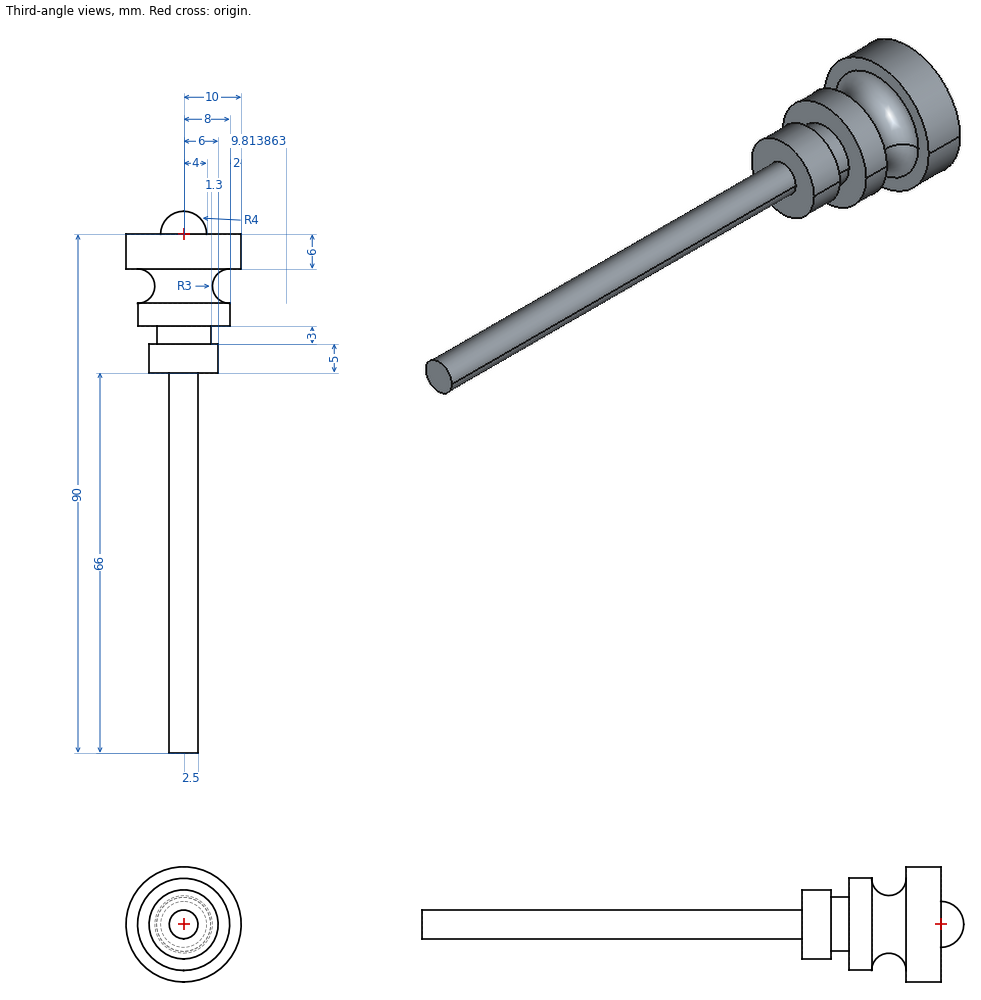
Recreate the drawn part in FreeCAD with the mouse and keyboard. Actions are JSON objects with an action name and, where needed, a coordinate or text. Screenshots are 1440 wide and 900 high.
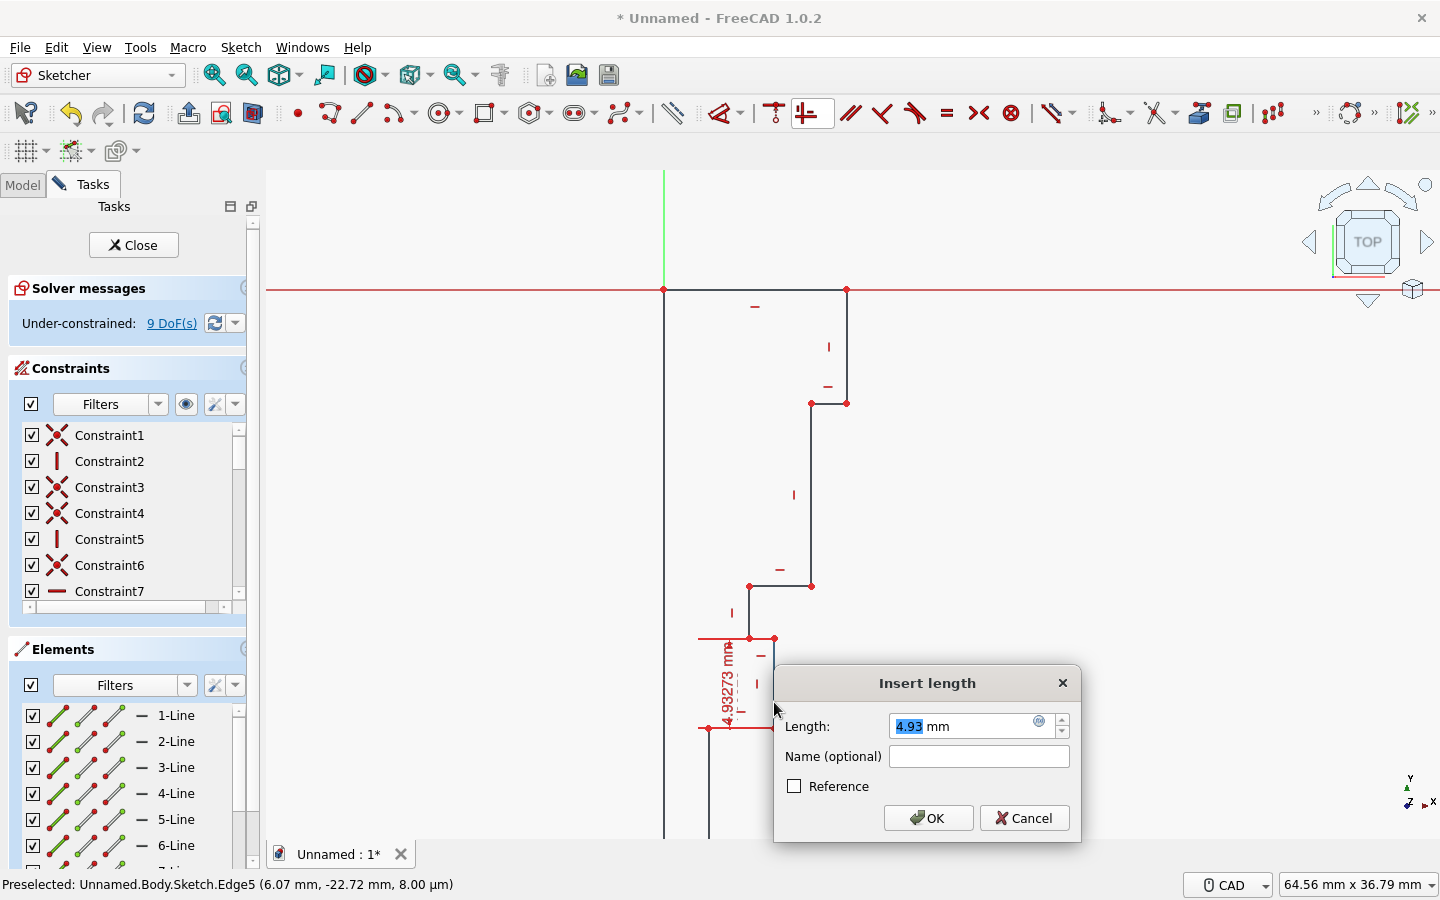
{"action": "type", "text": "5"}
{"action": "key", "text": "Return"}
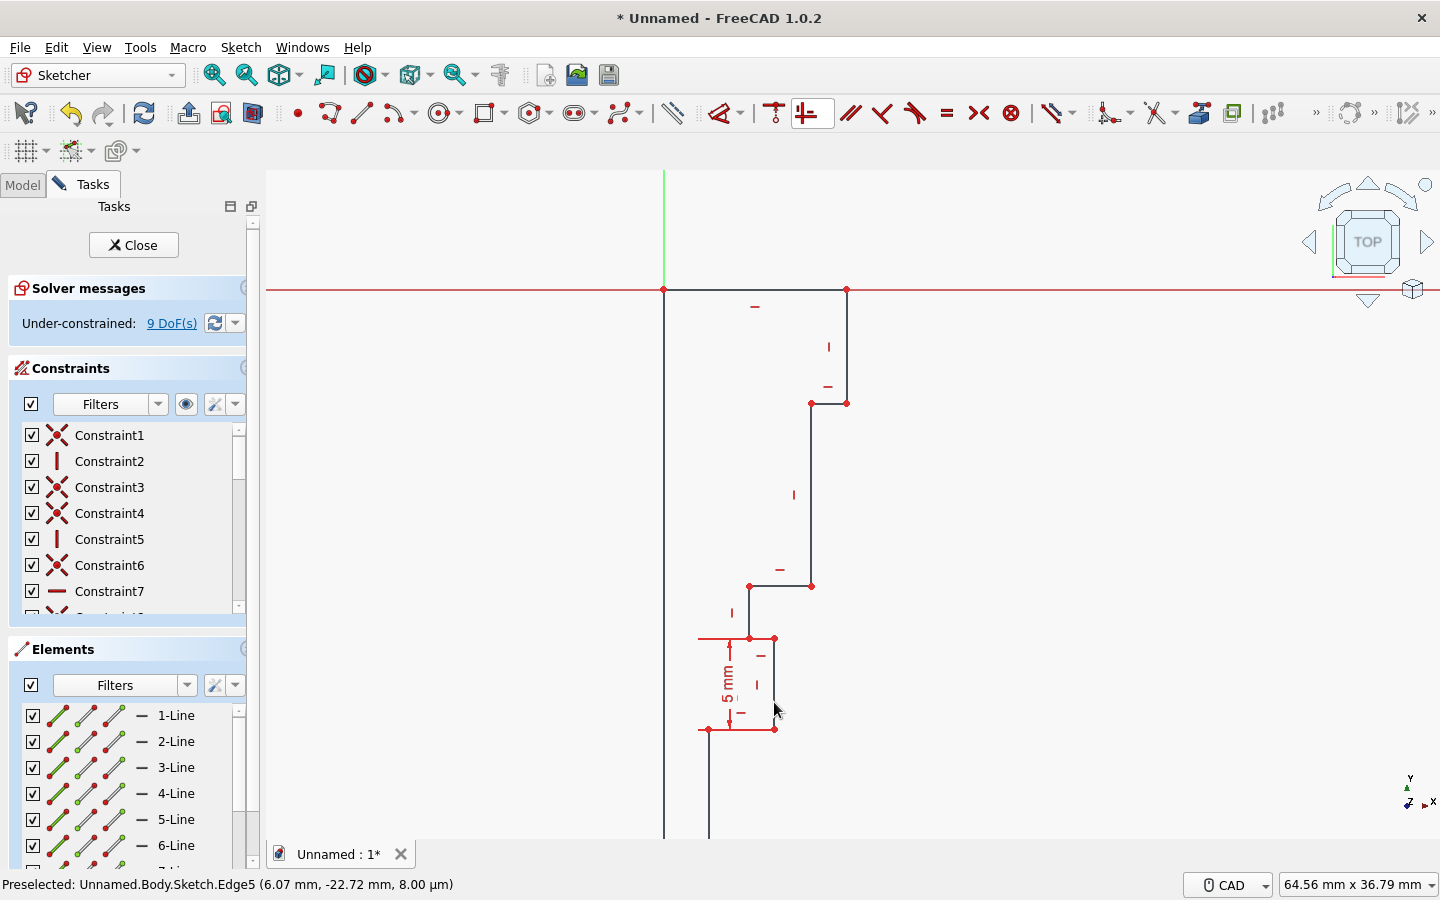
{"action": "left_click", "coordinate": [749, 623]}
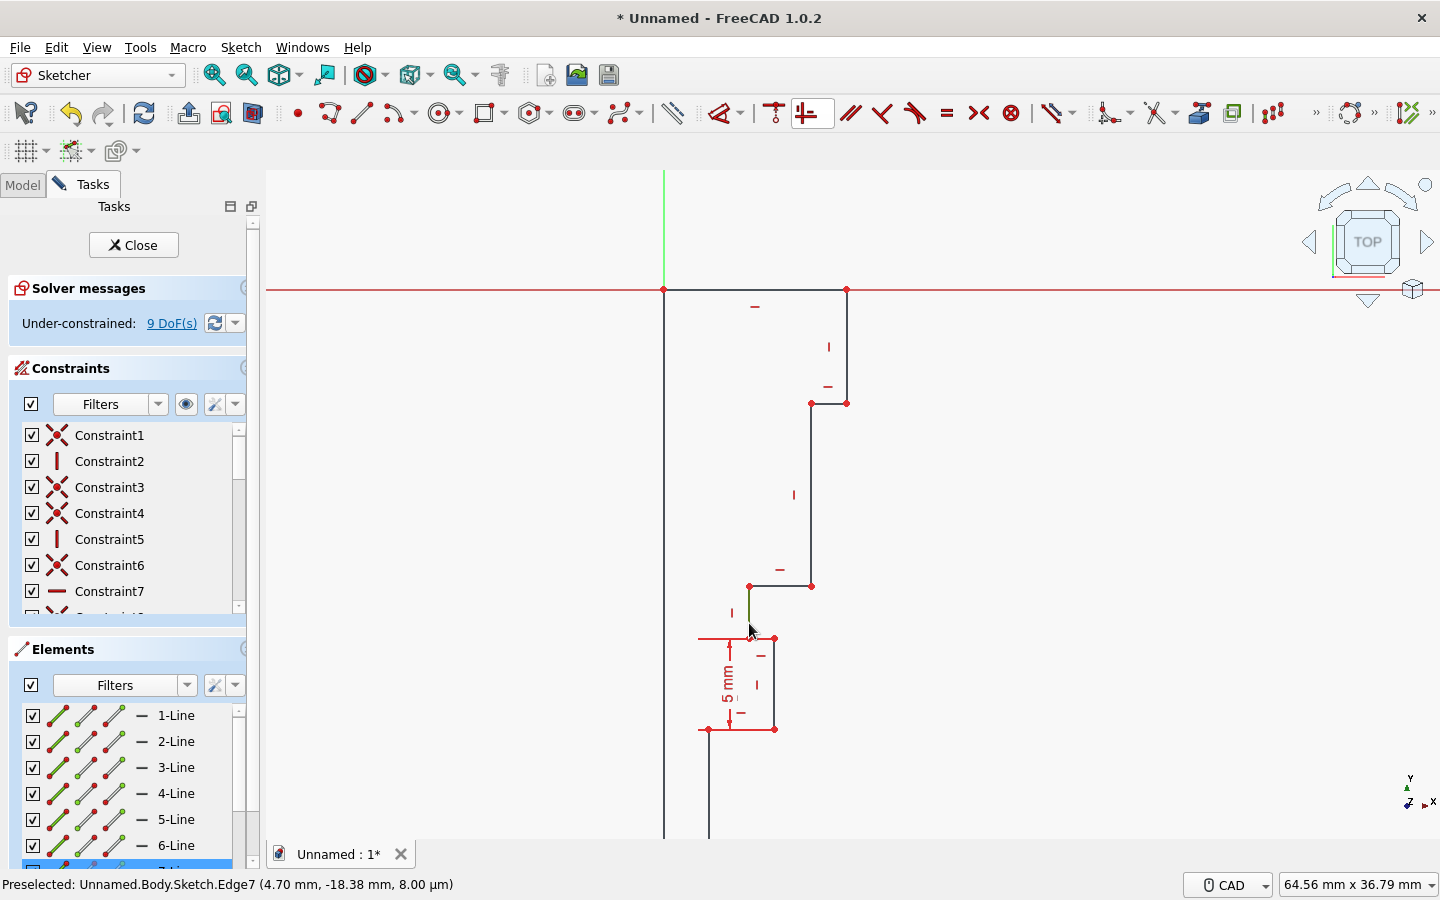
{"action": "key", "text": "i"}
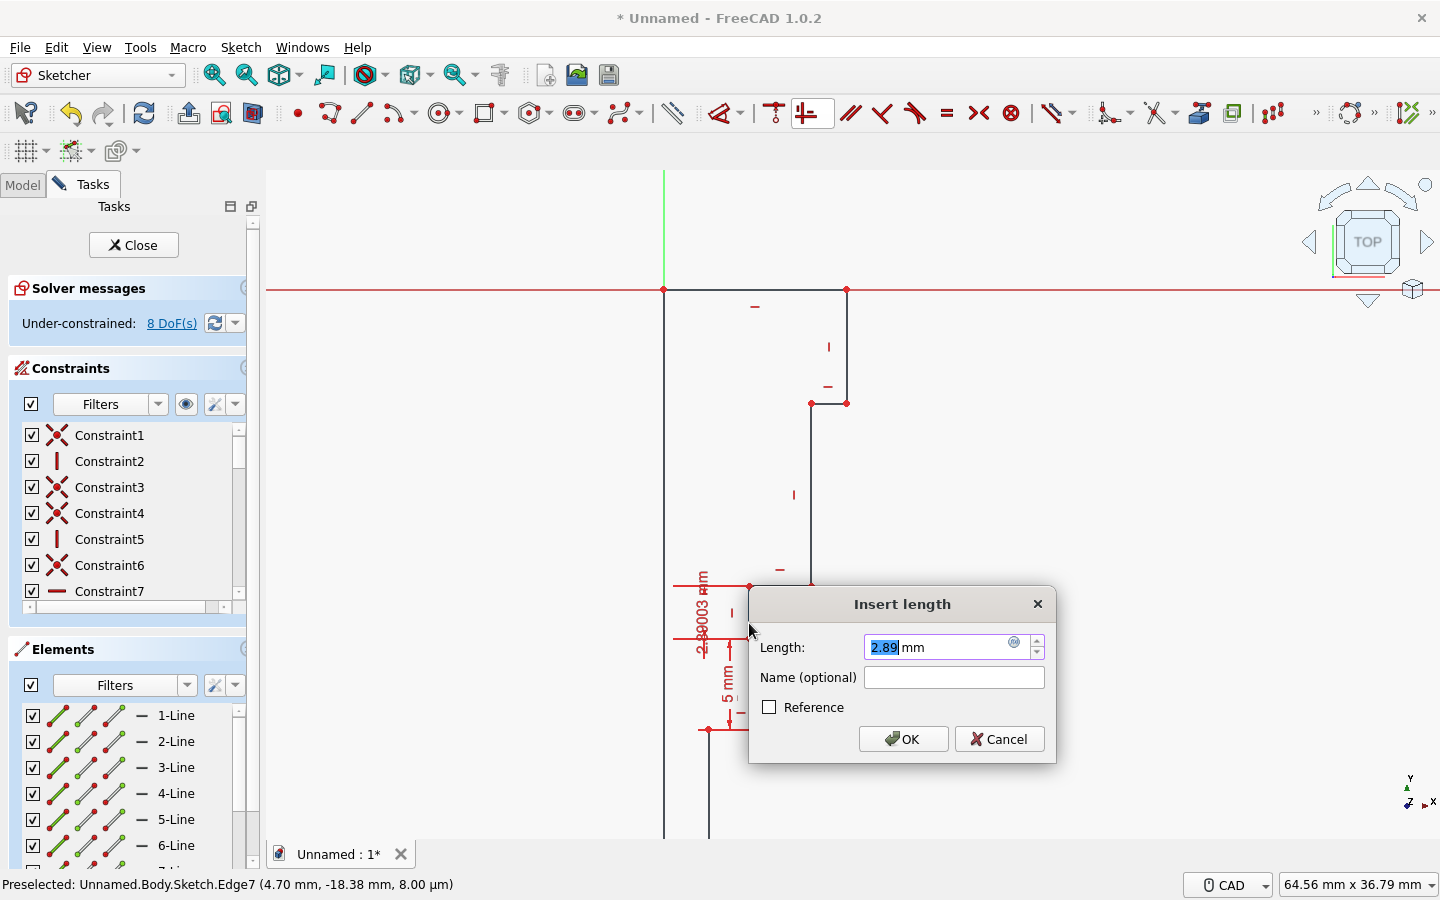
{"action": "type", "text": "3"}
{"action": "key", "text": "Return"}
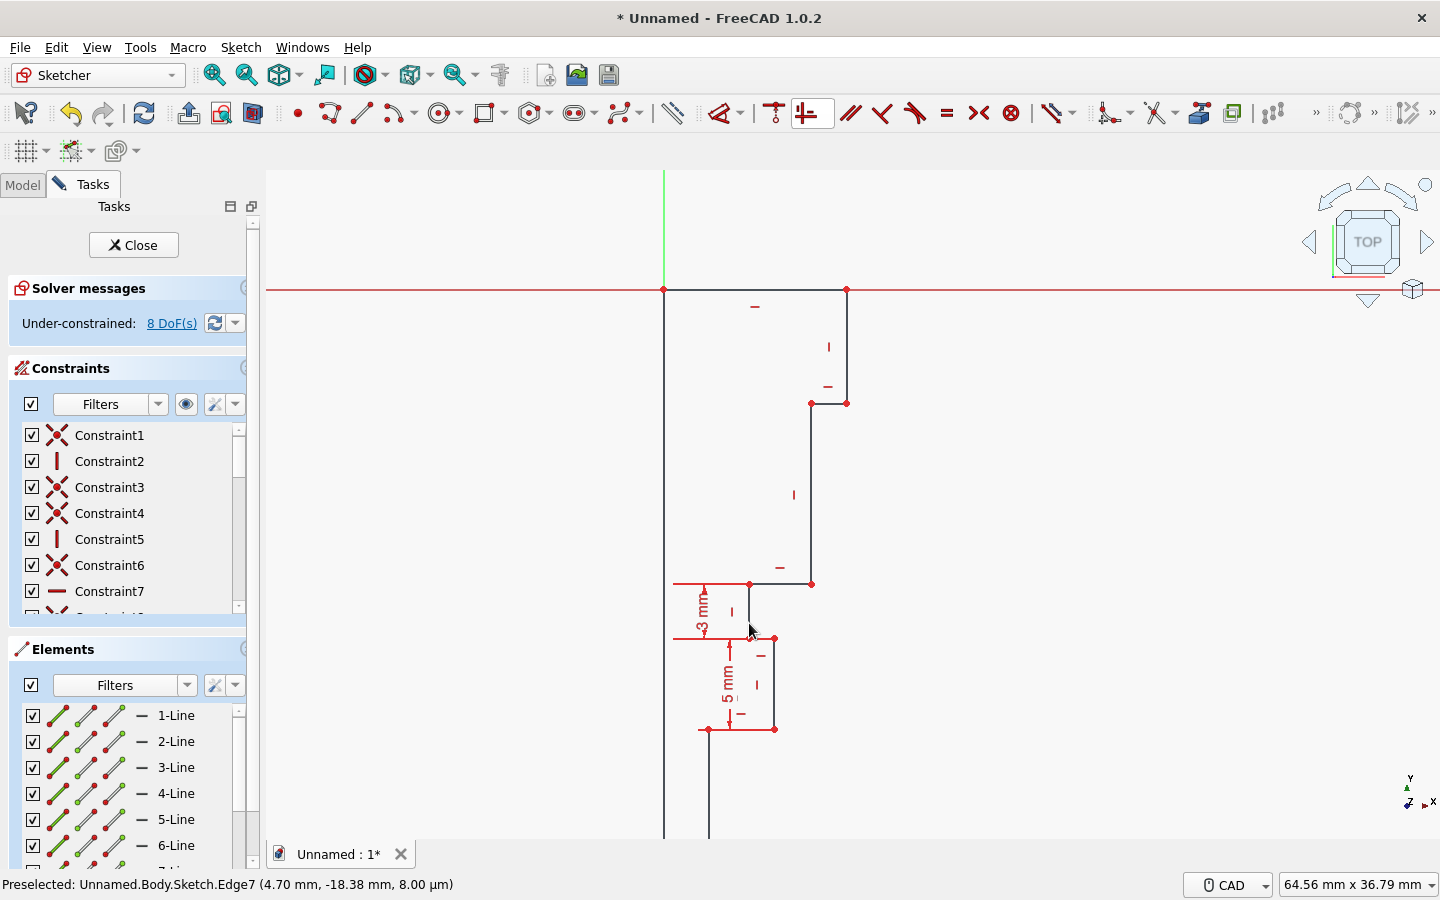
{"action": "scroll", "coordinate": [822, 404], "scroll_direction": "up", "scroll_amount": 2}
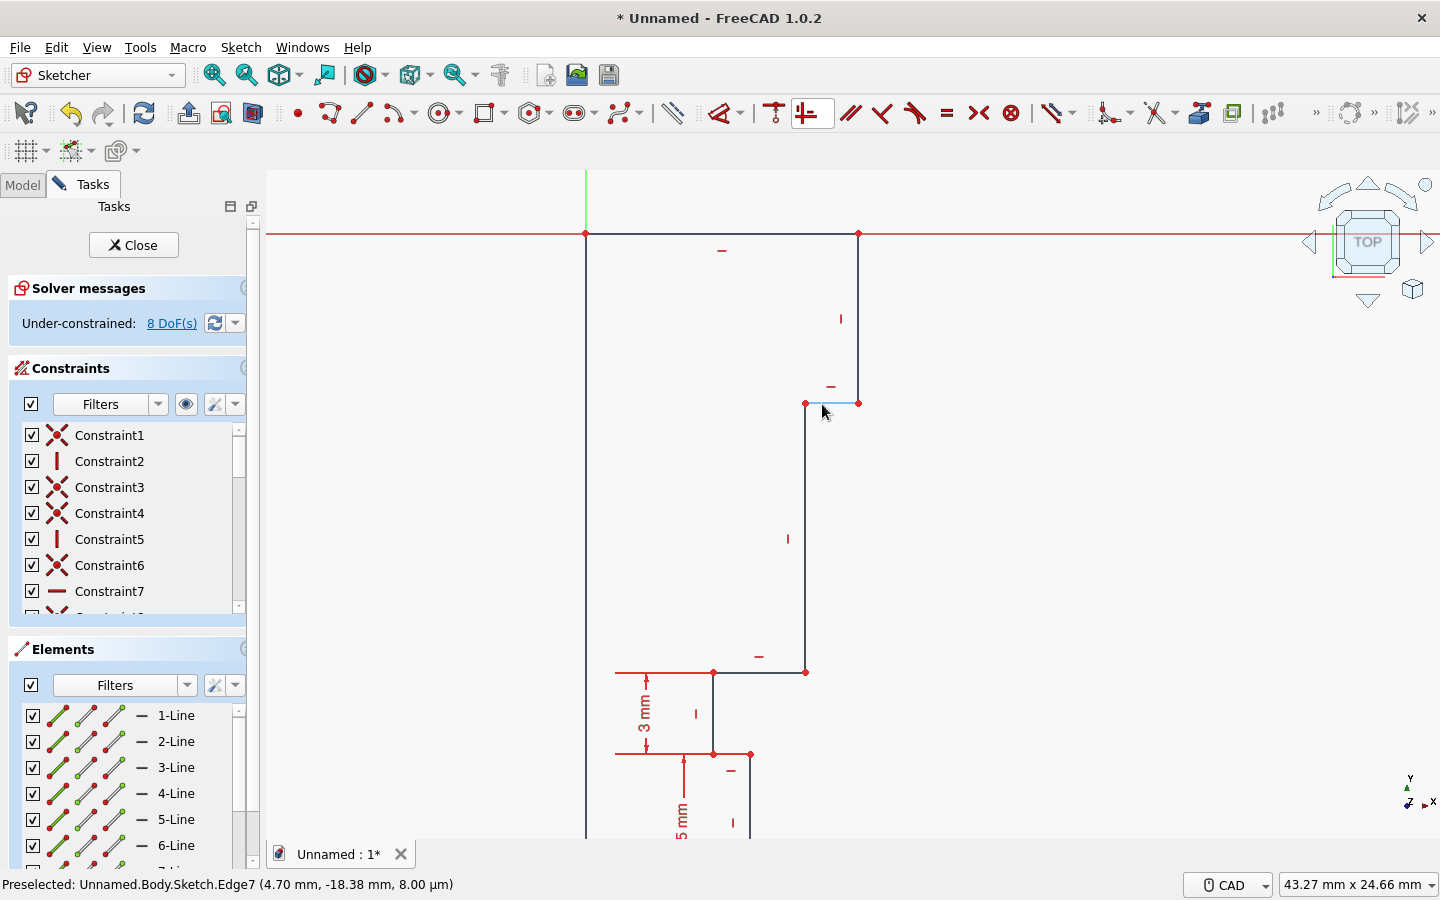
{"action": "left_click", "coordinate": [821, 403]}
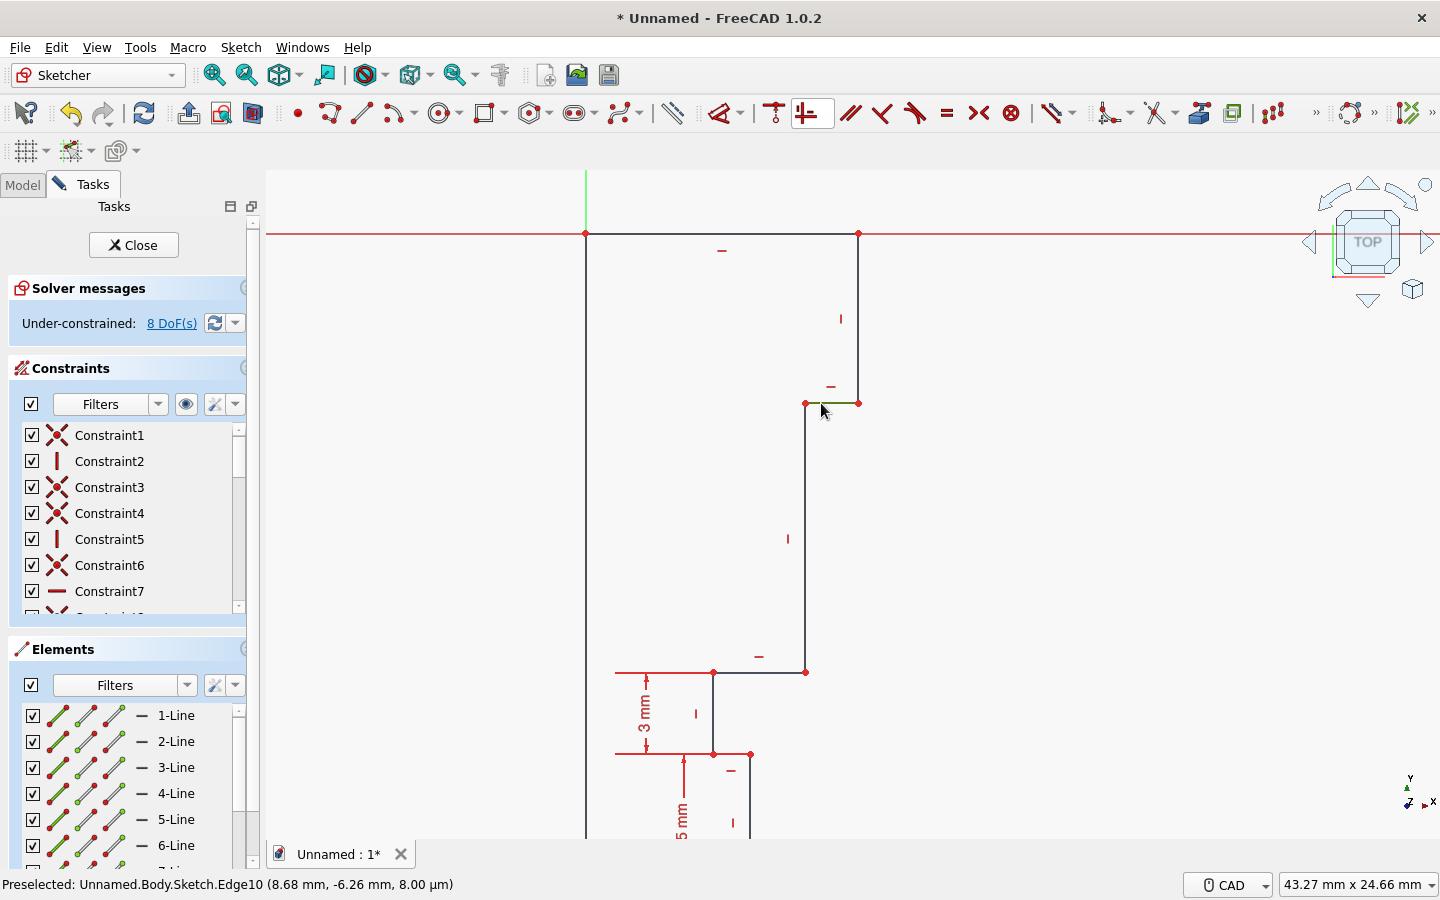
{"action": "key", "text": "l"}